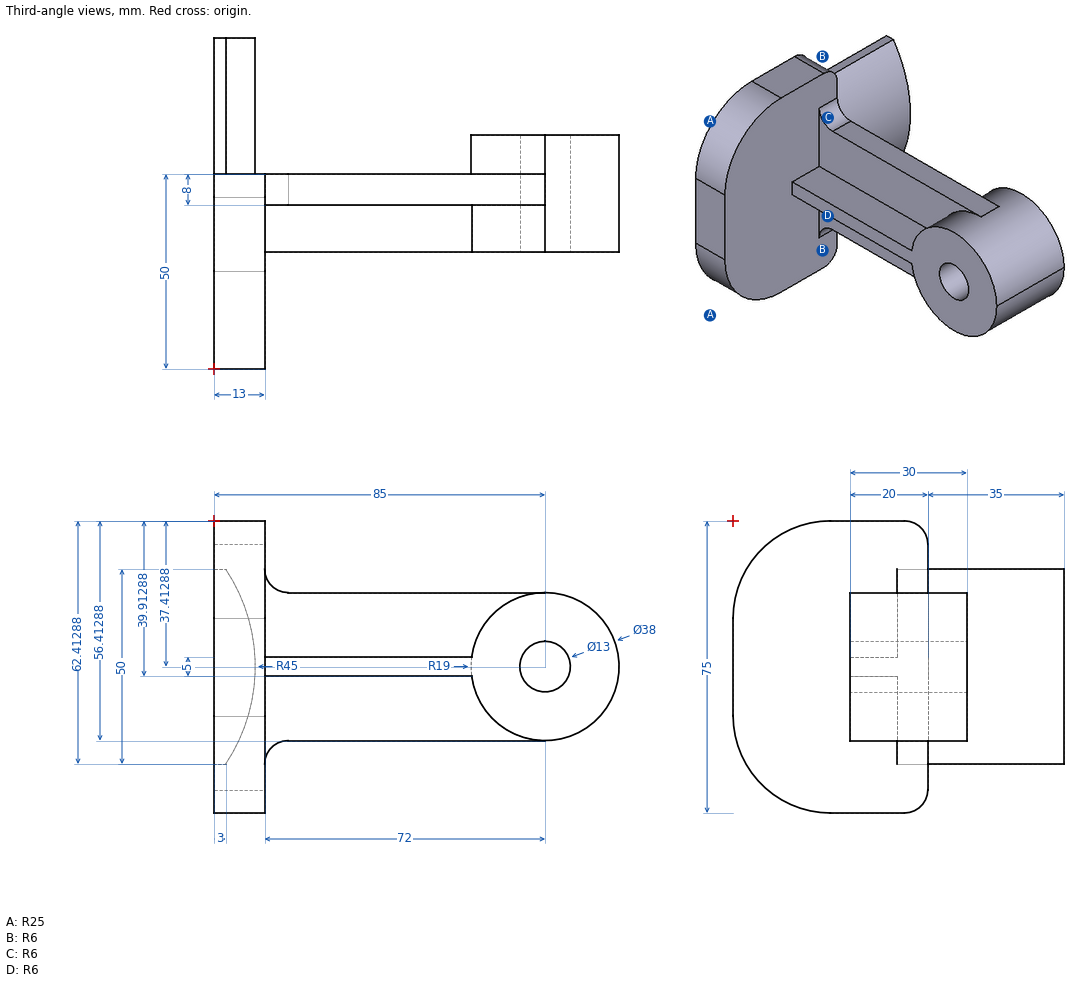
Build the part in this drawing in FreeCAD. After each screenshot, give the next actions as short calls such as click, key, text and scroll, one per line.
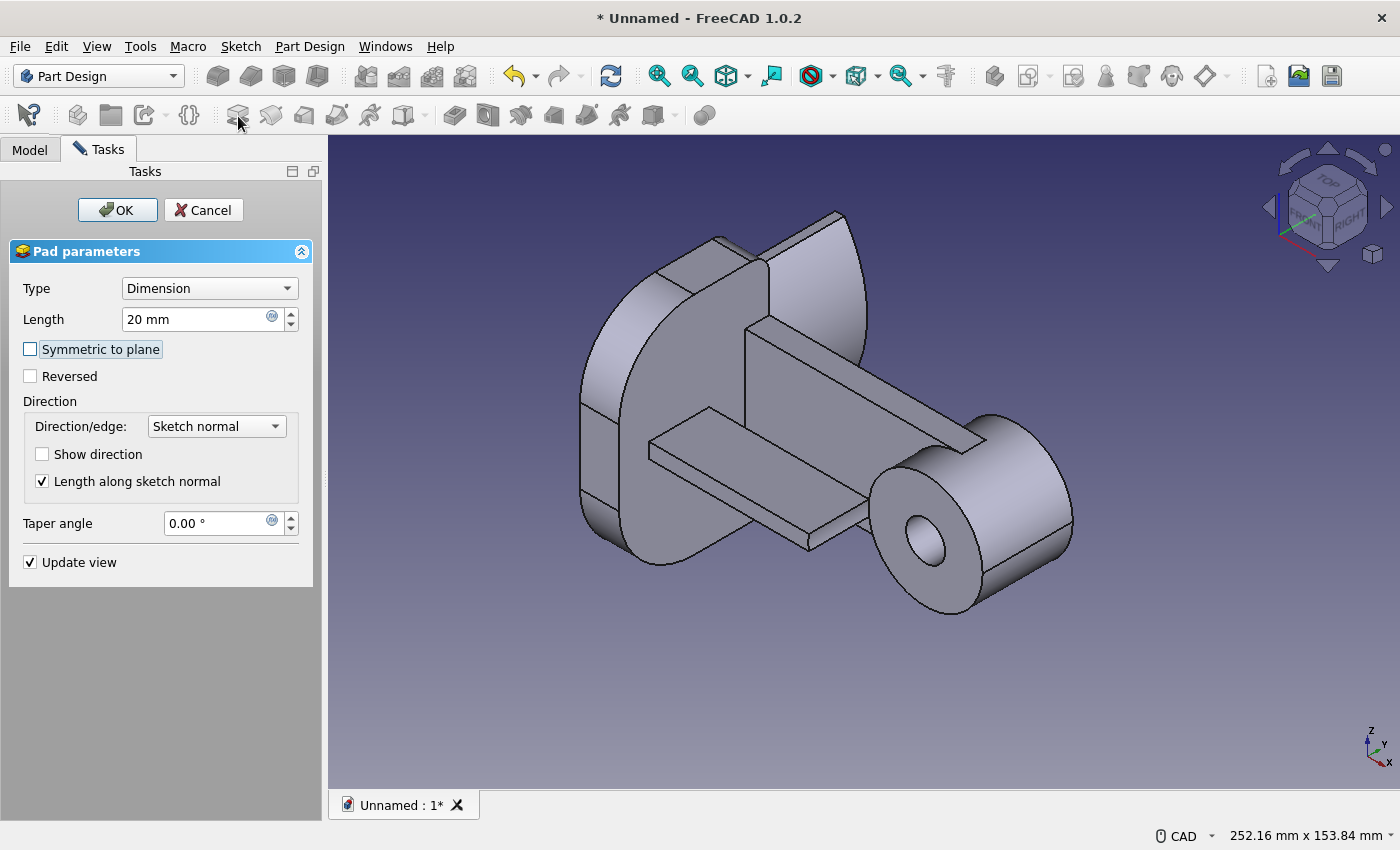
click(31, 376)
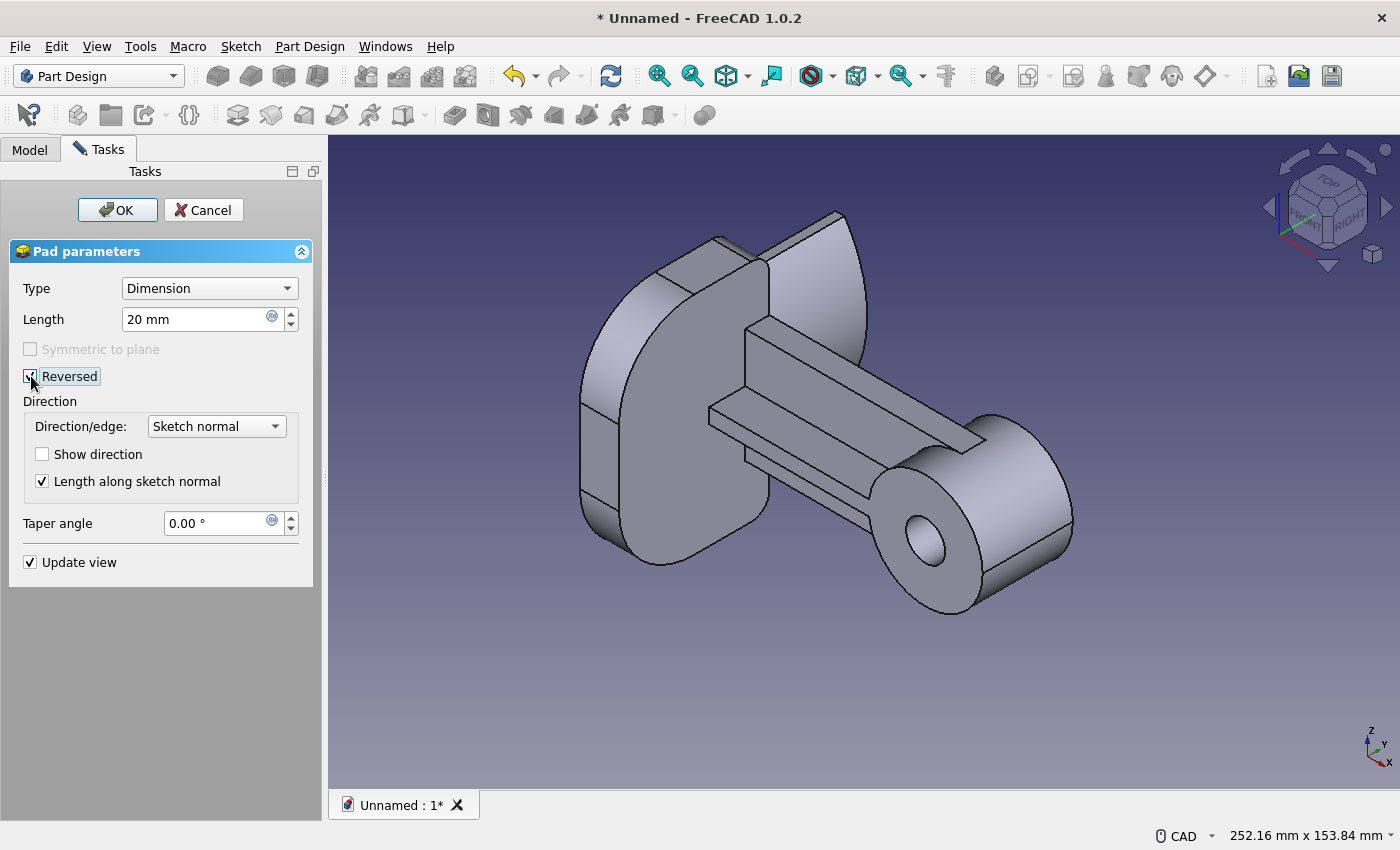
click(118, 210)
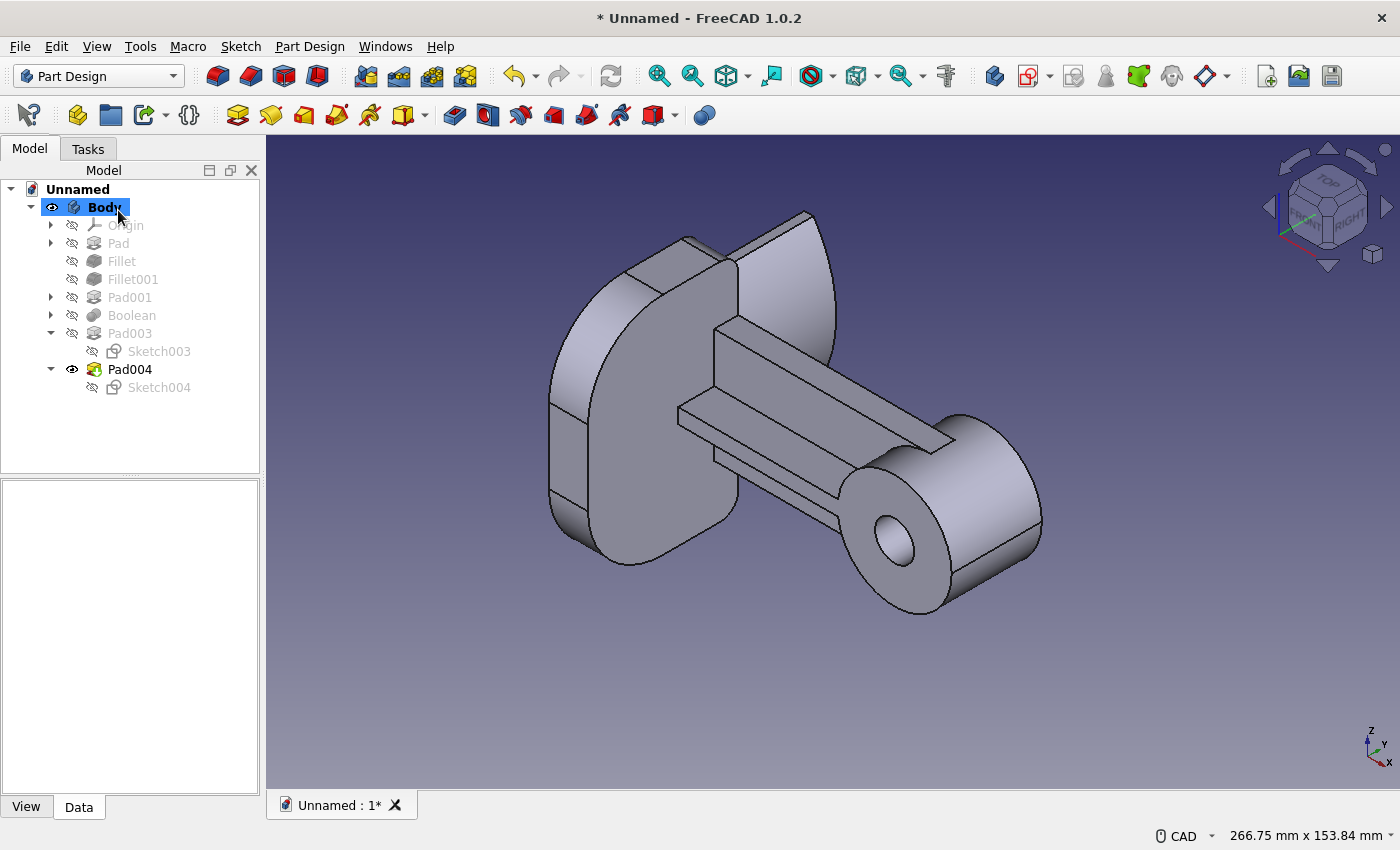
key(2)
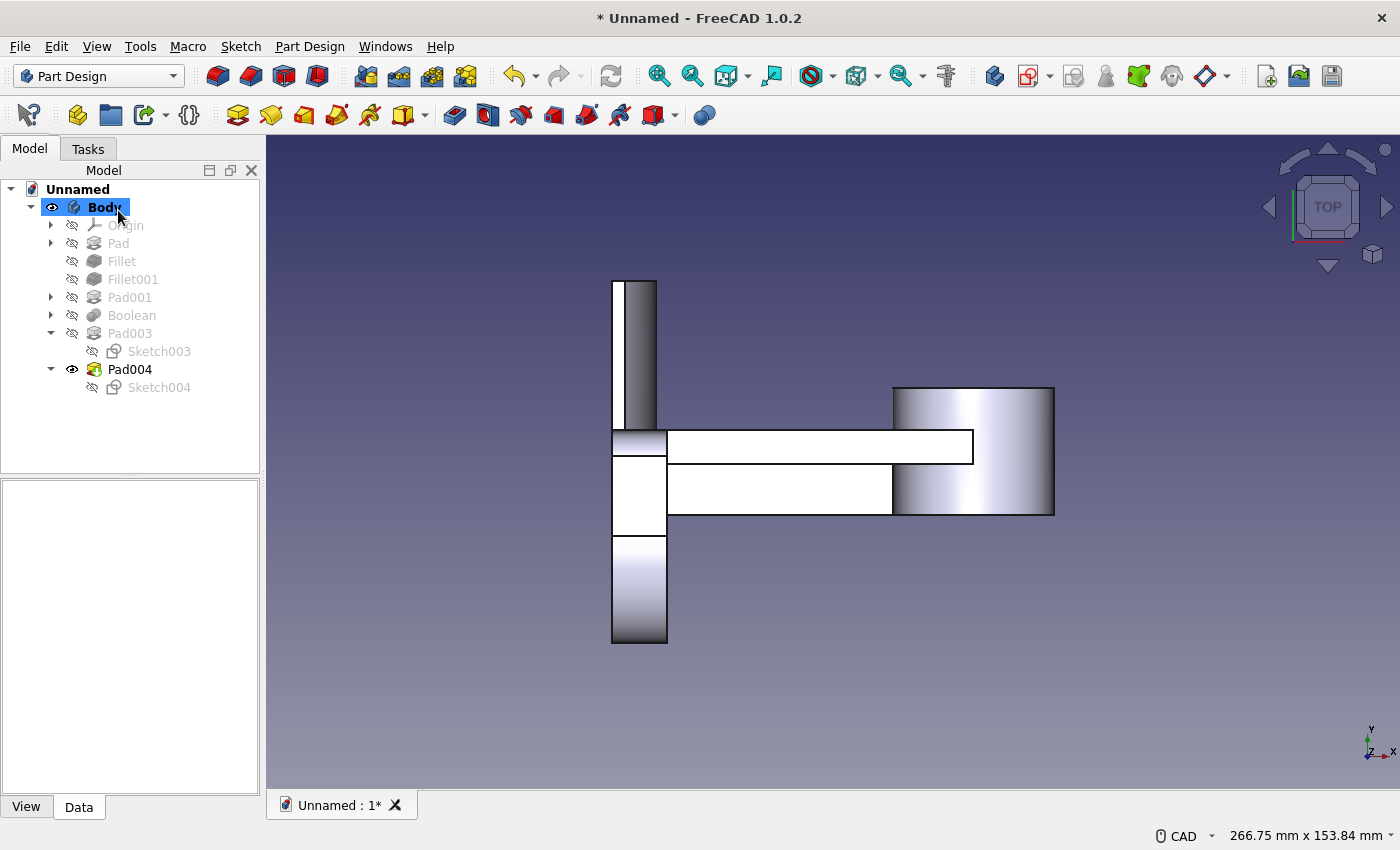
key(0)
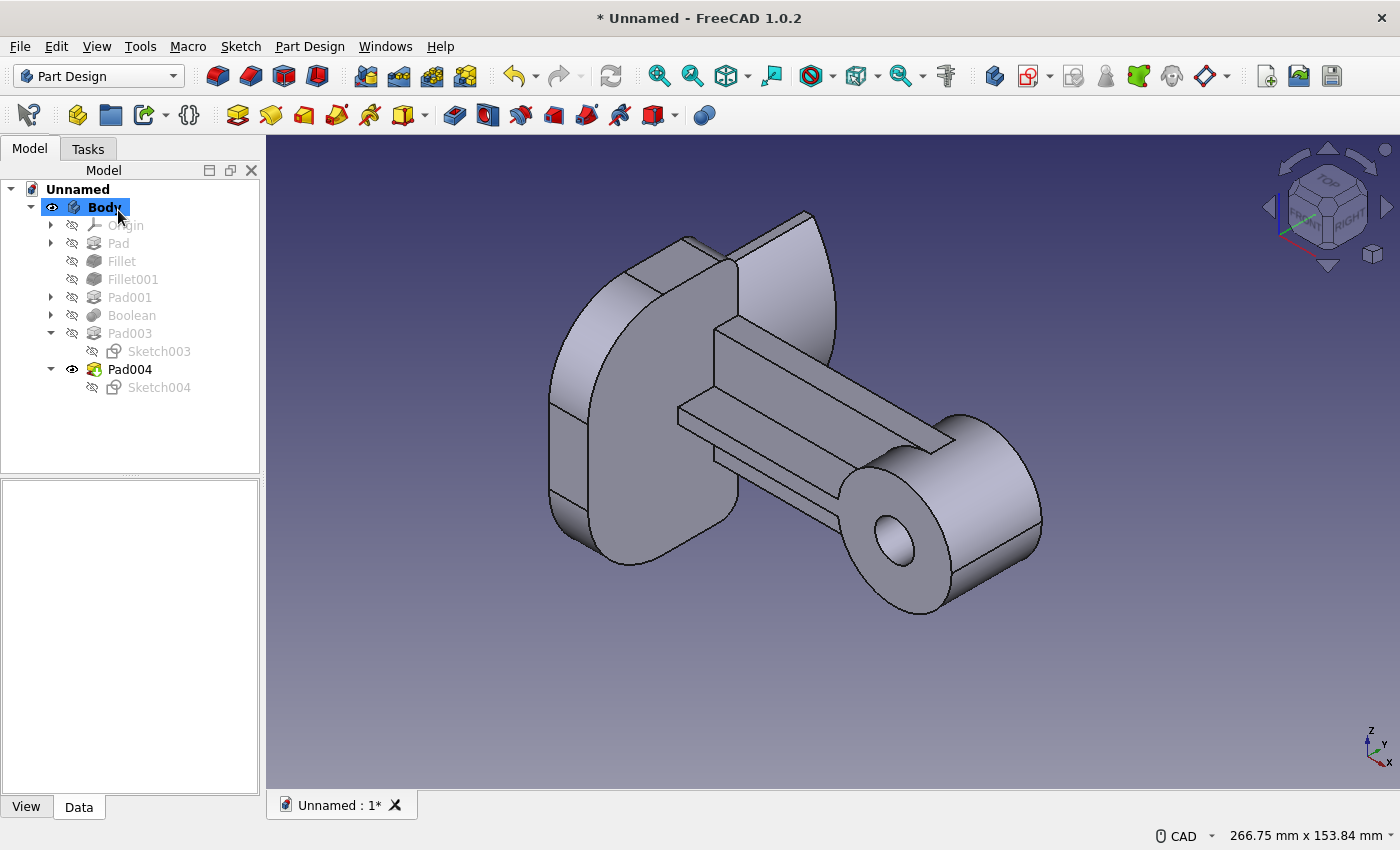
key(1)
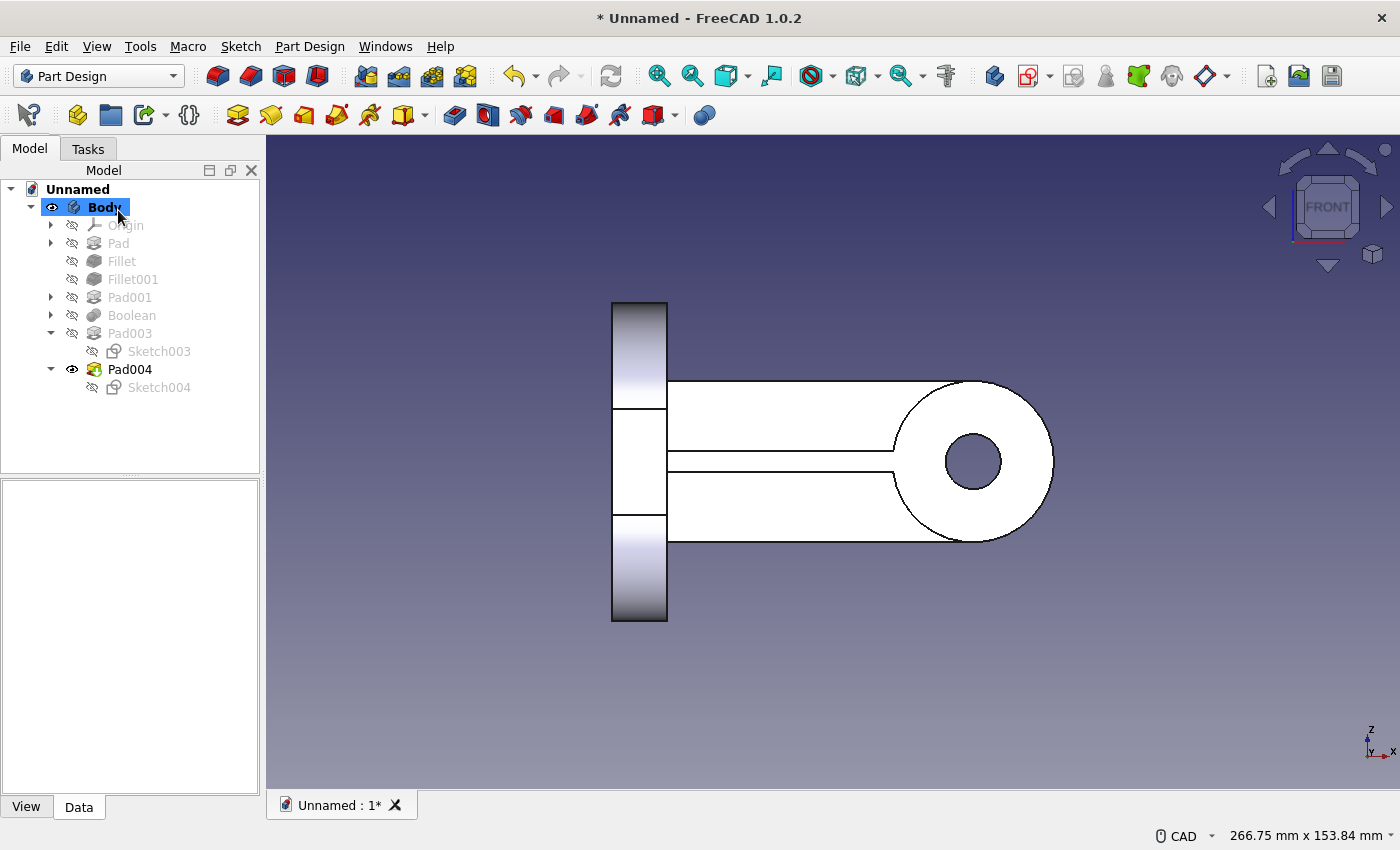
key(3)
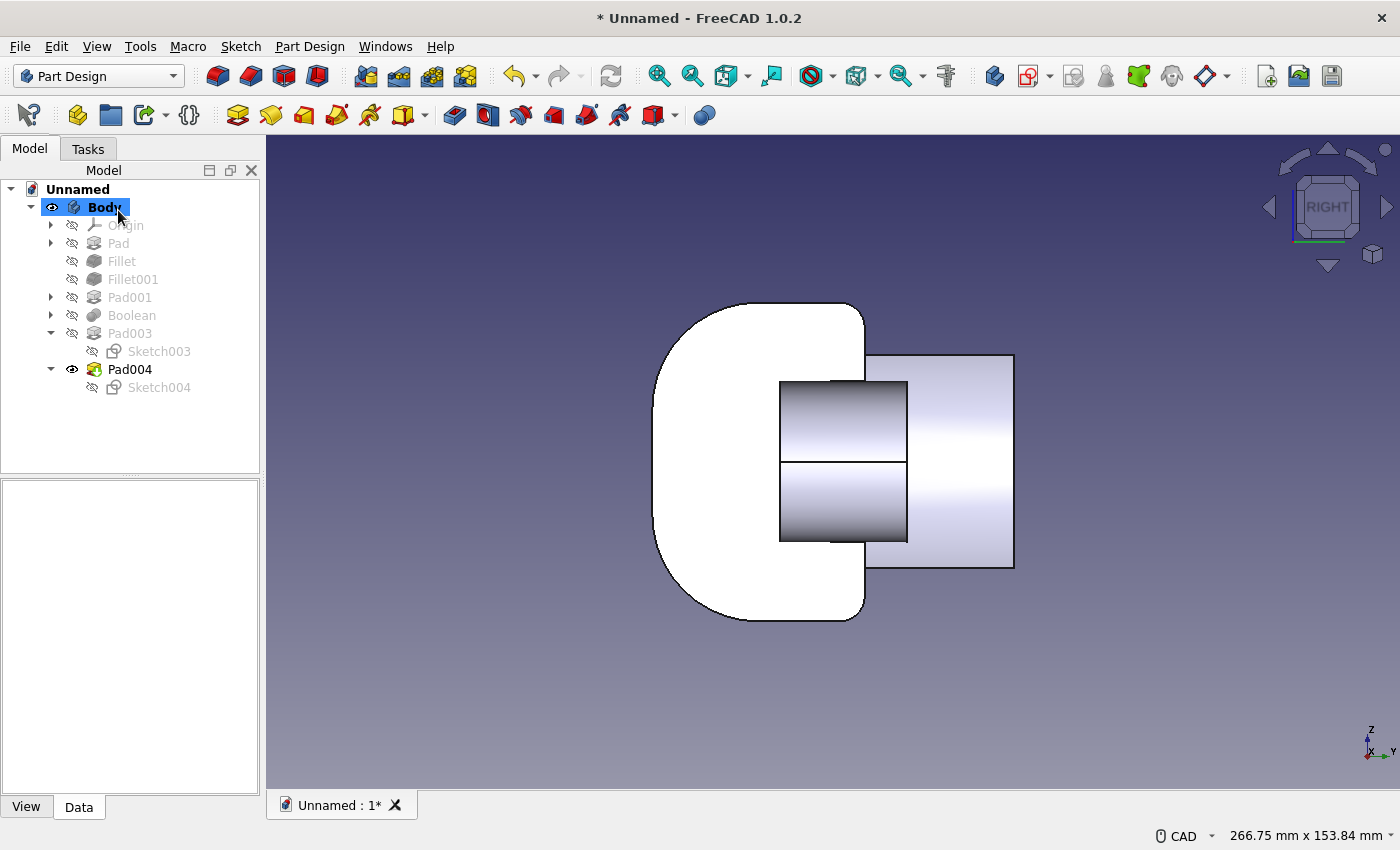
key(5)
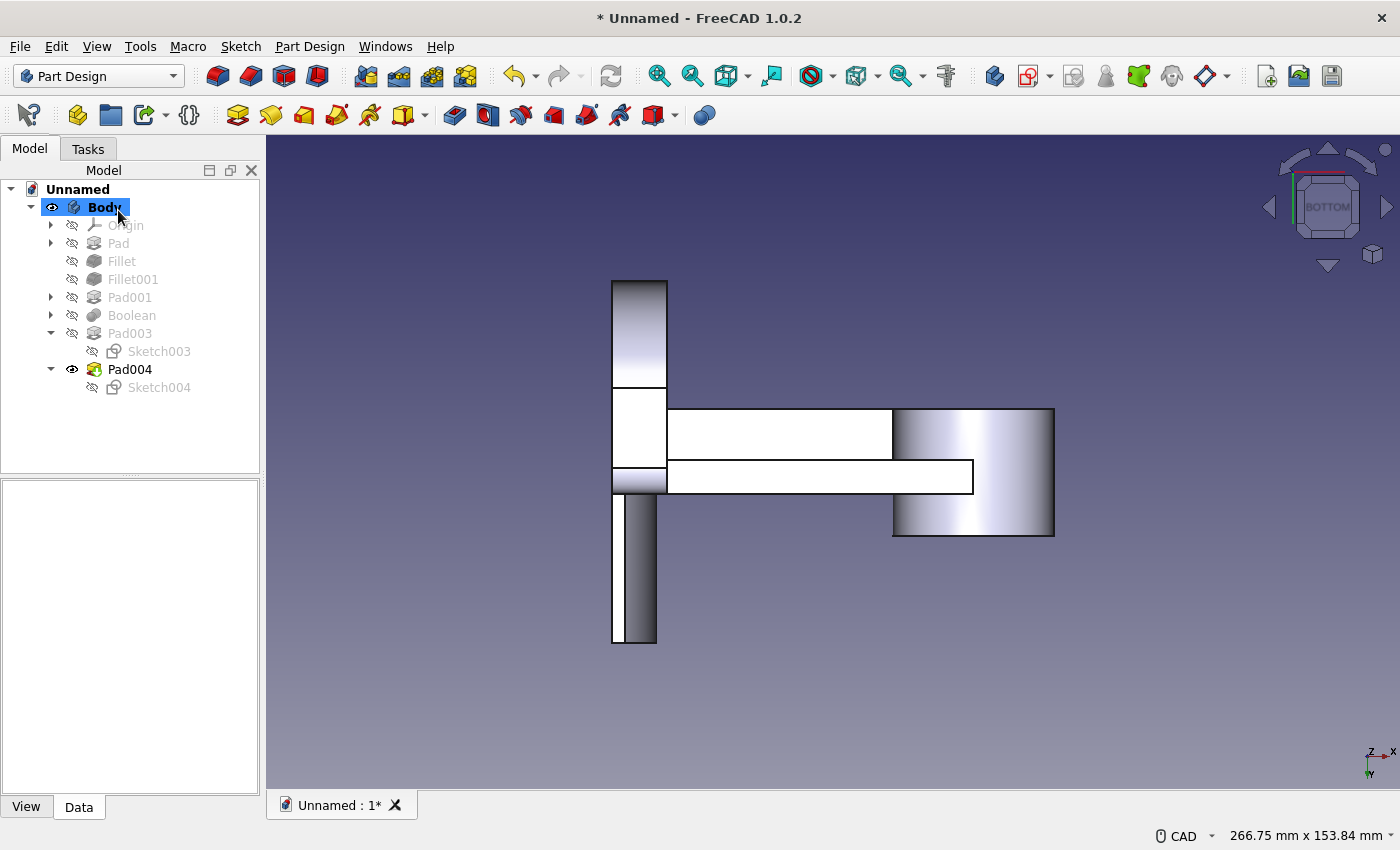
key(4)